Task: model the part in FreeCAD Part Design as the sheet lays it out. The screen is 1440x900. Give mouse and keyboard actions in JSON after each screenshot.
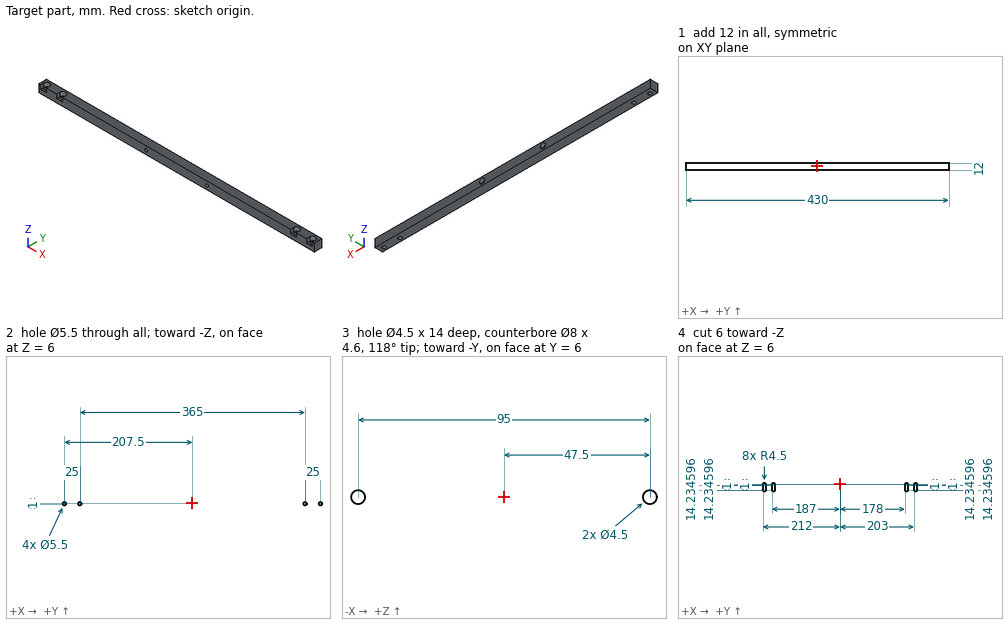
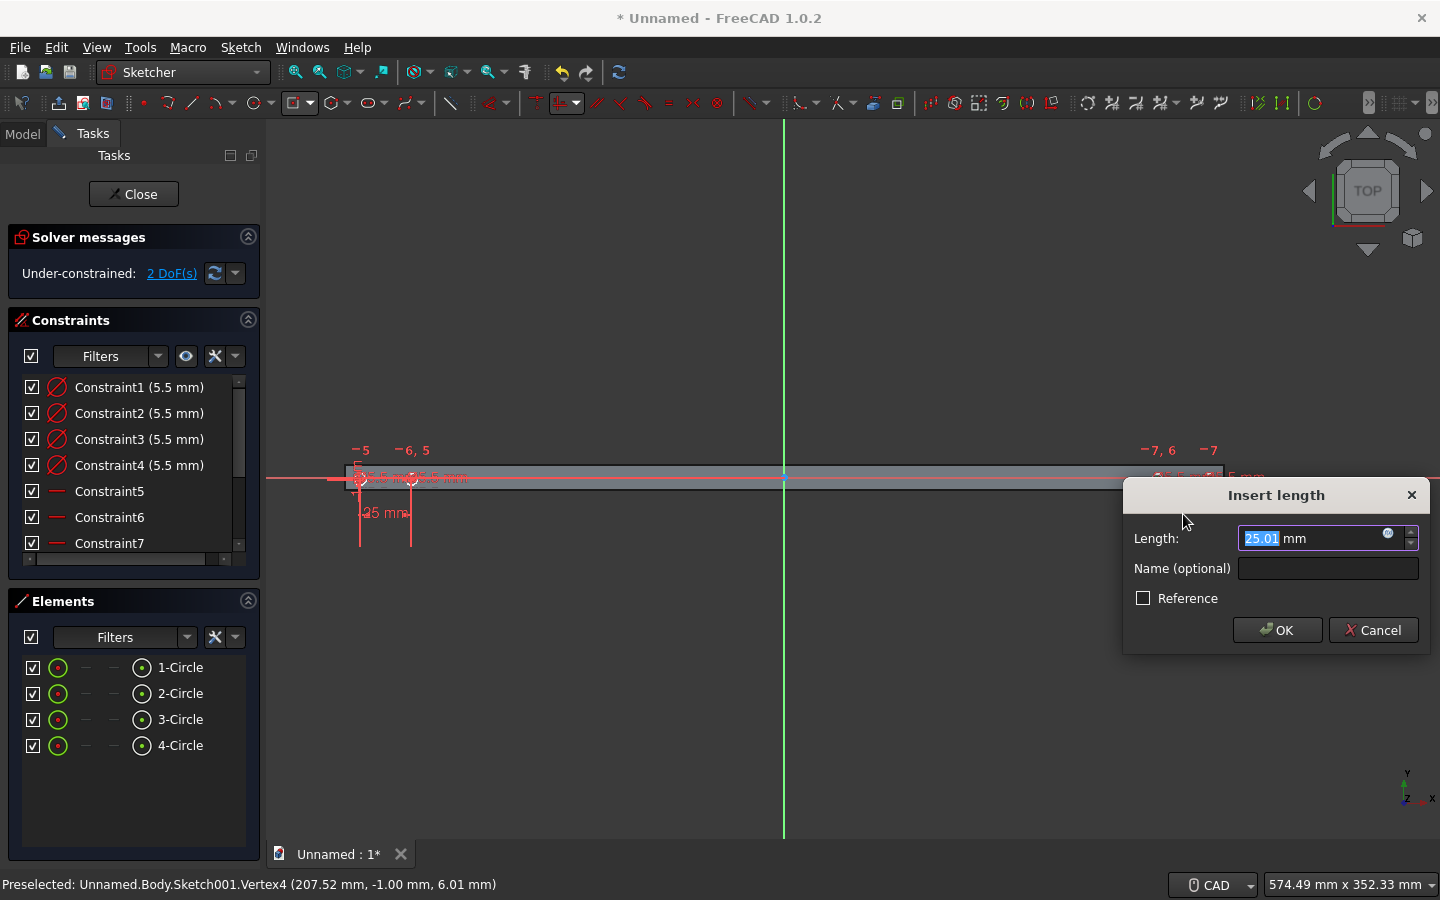
{"action": "type", "text": "25"}
{"action": "key", "text": "Return"}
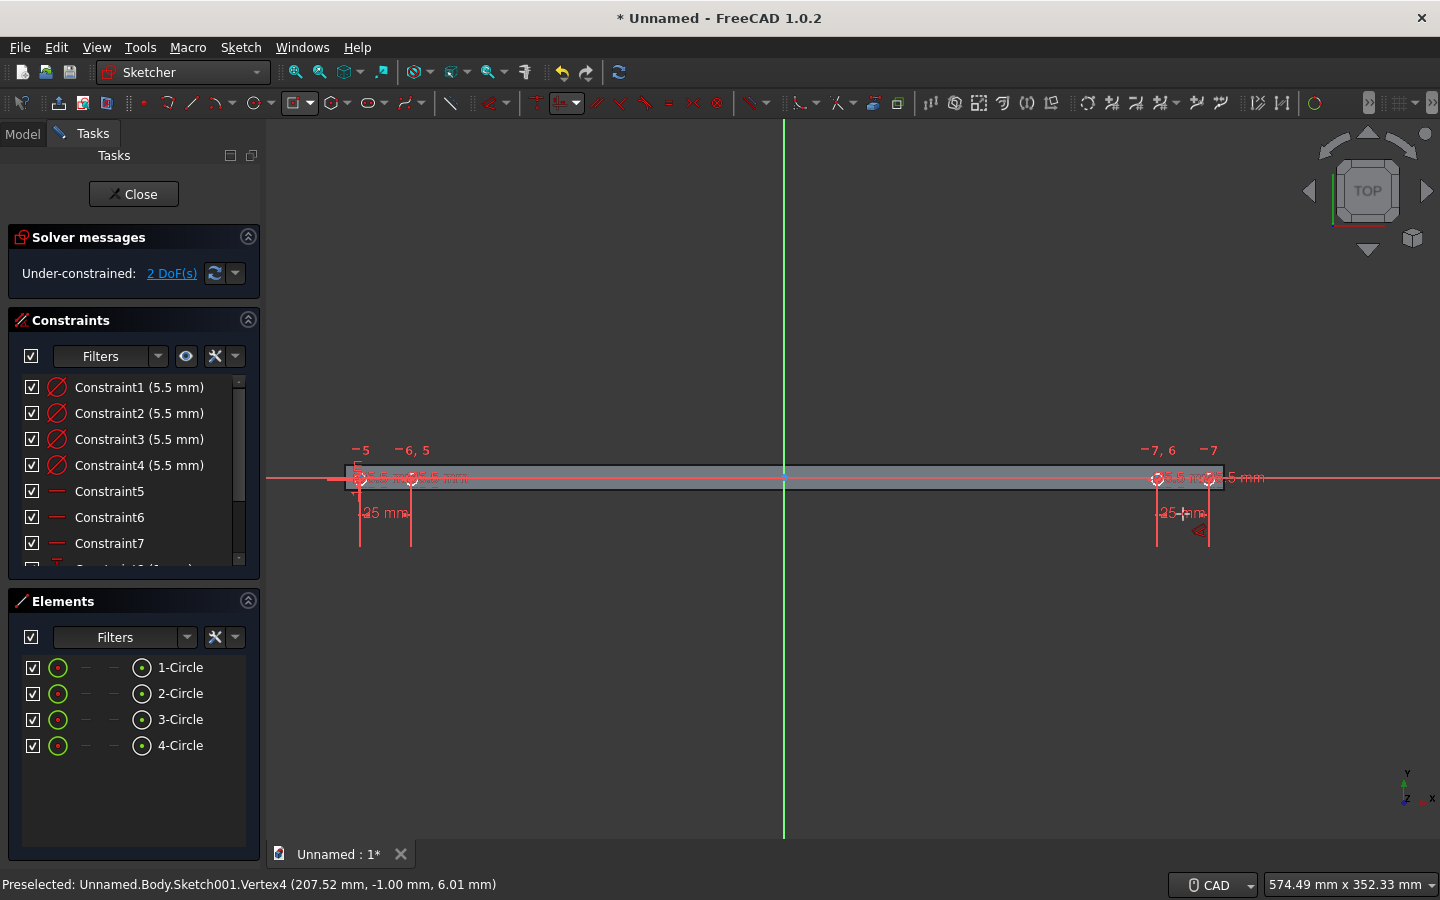
{"action": "left_click", "coordinate": [411, 480]}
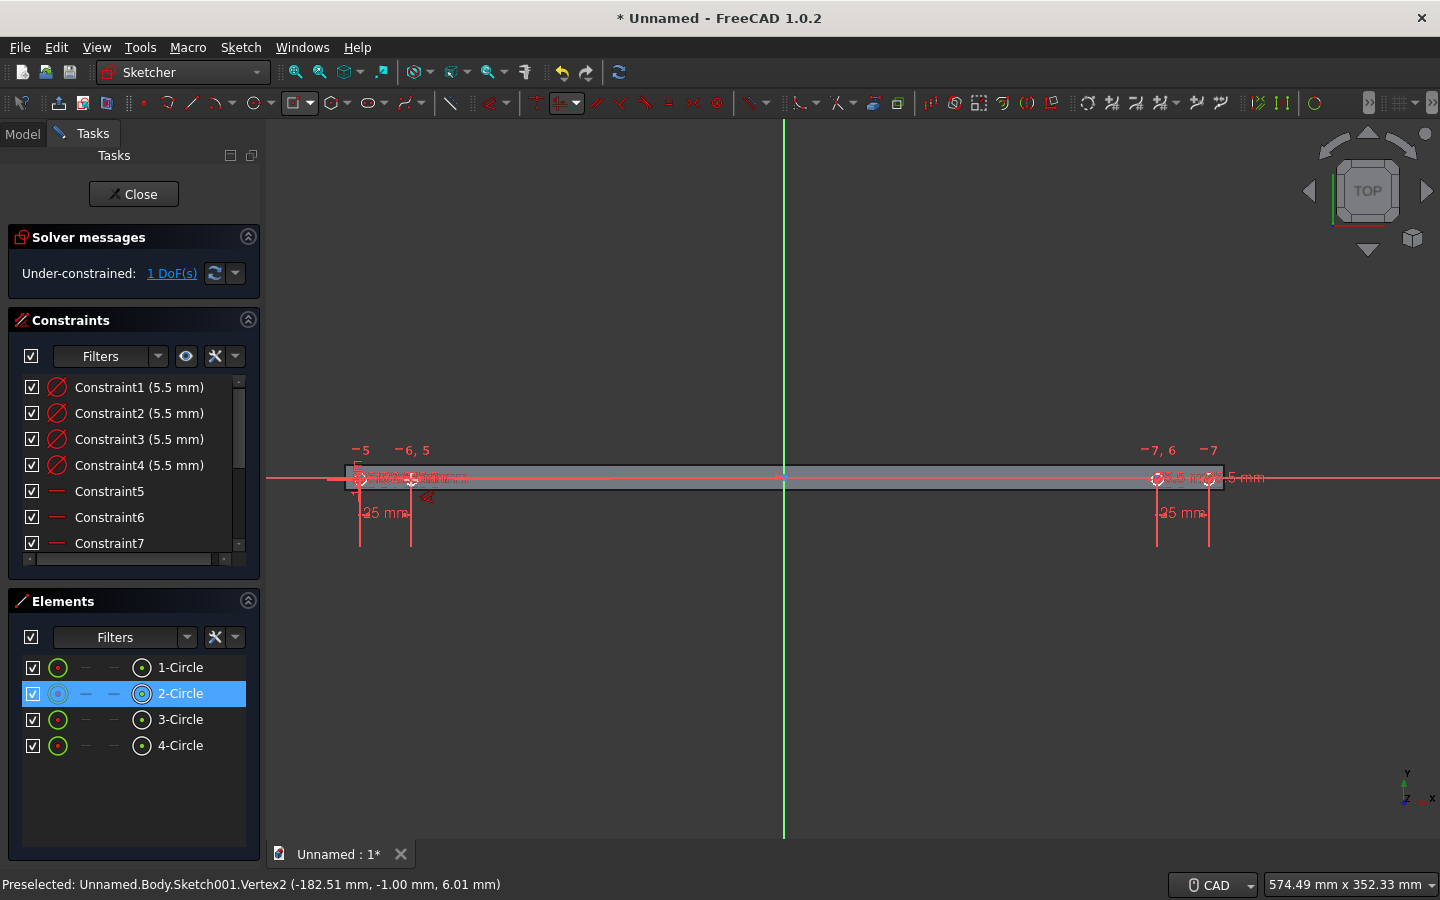
{"action": "left_click", "coordinate": [1157, 480]}
{"action": "left_click", "coordinate": [613, 514]}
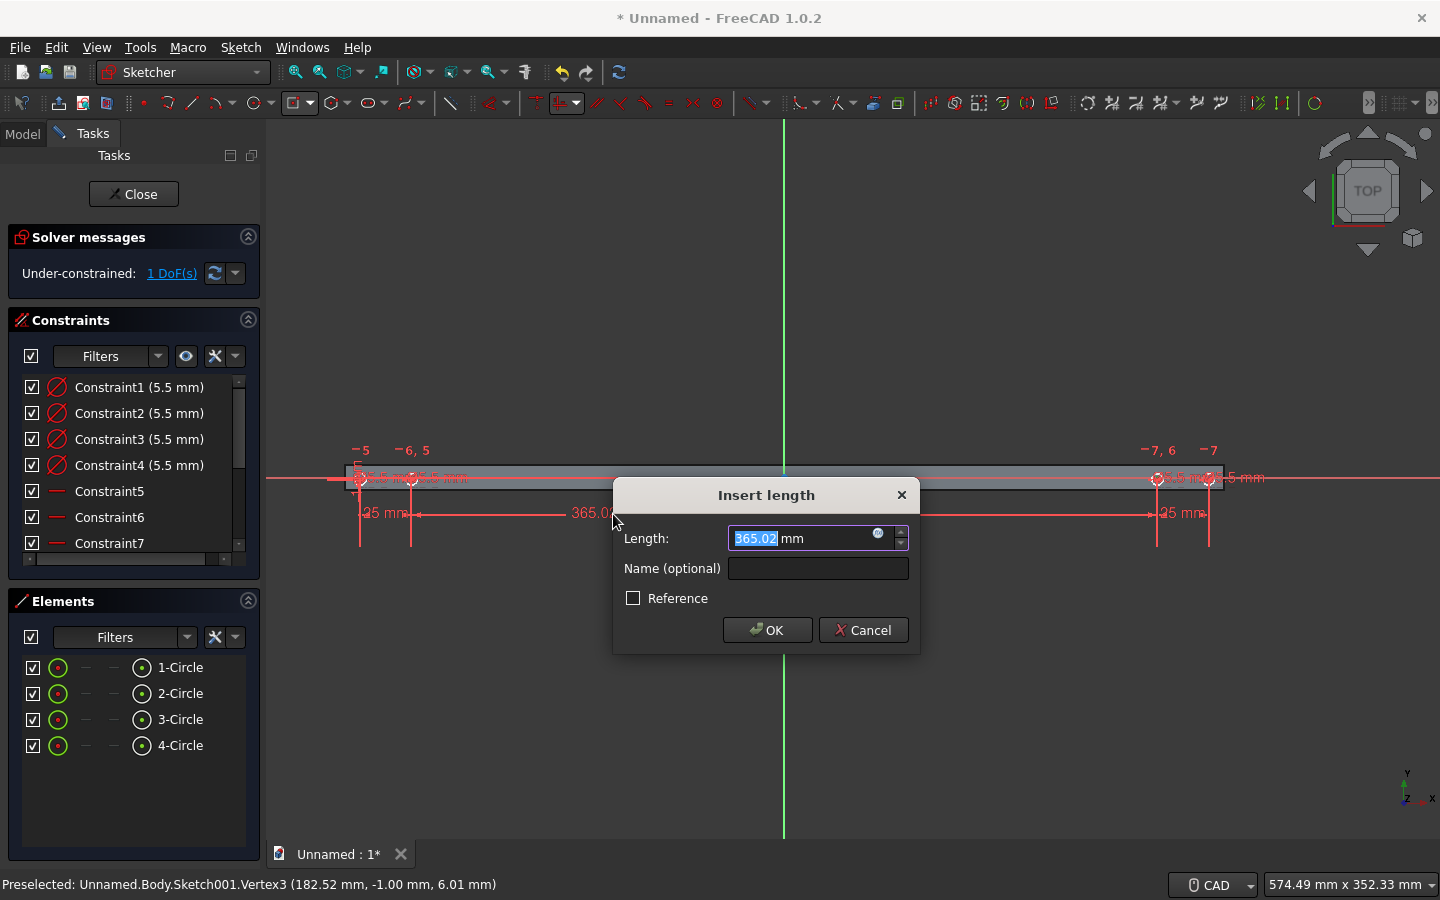
{"action": "type", "text": "365"}
{"action": "key", "text": "Return"}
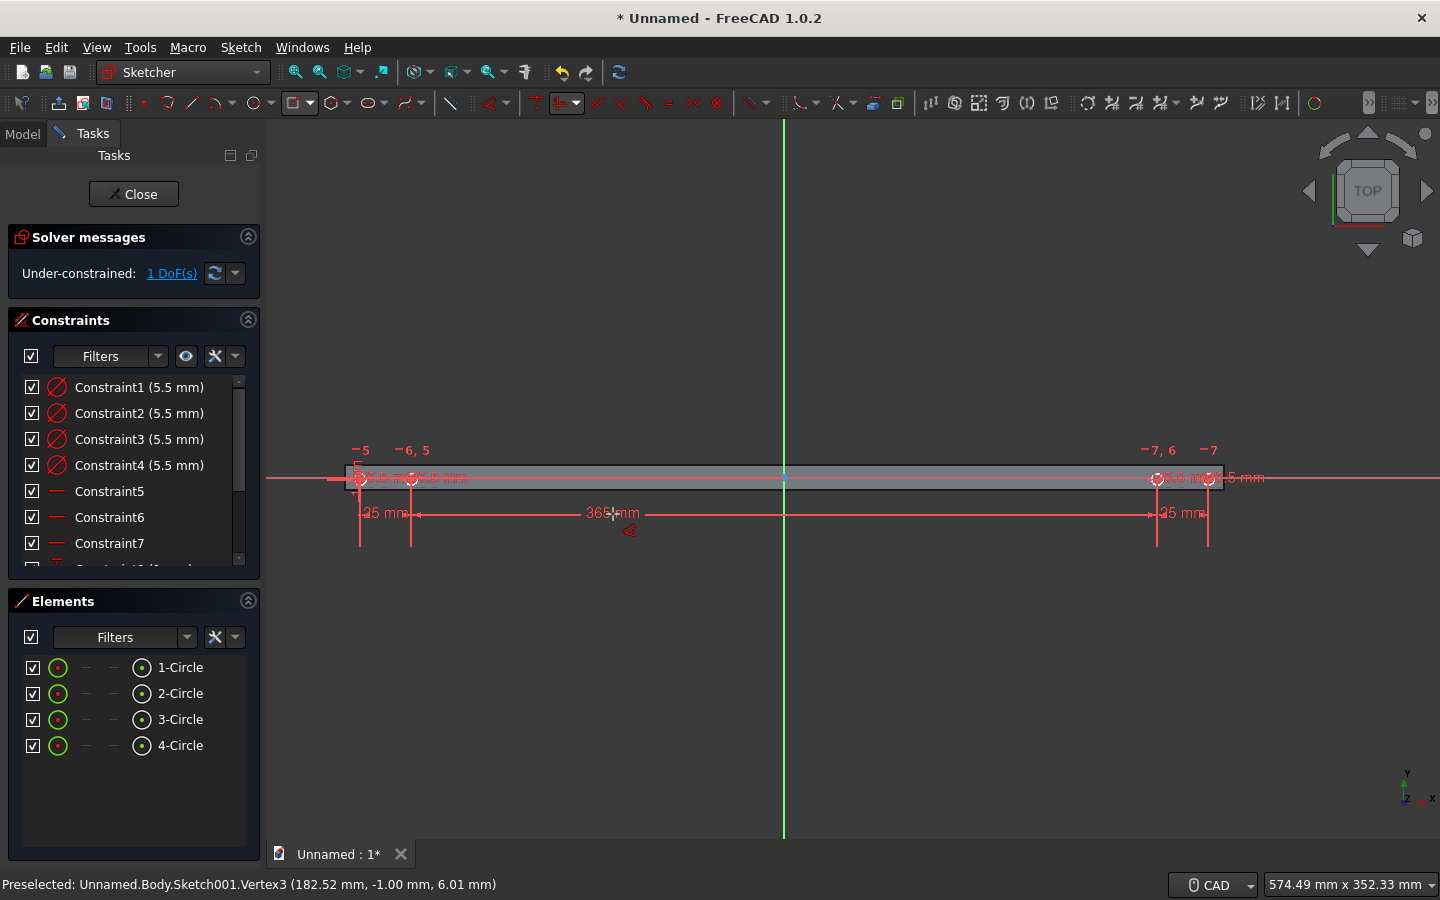
{"action": "left_click", "coordinate": [360, 480]}
{"action": "left_click", "coordinate": [572, 444]}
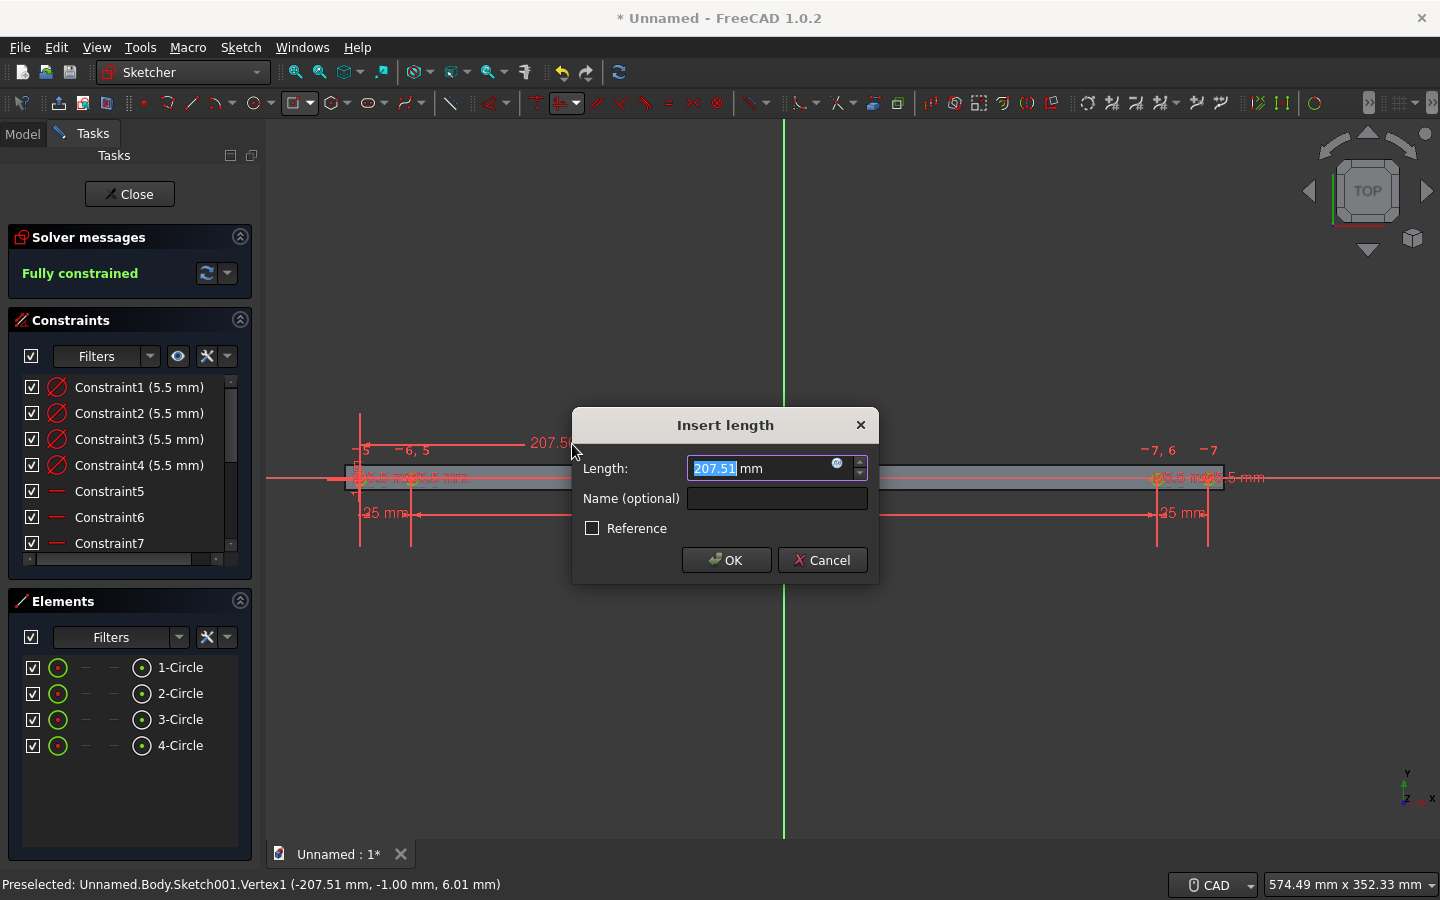
{"action": "type", "text": "207.5"}
{"action": "key", "text": "Return"}
{"action": "key", "text": "Escape"}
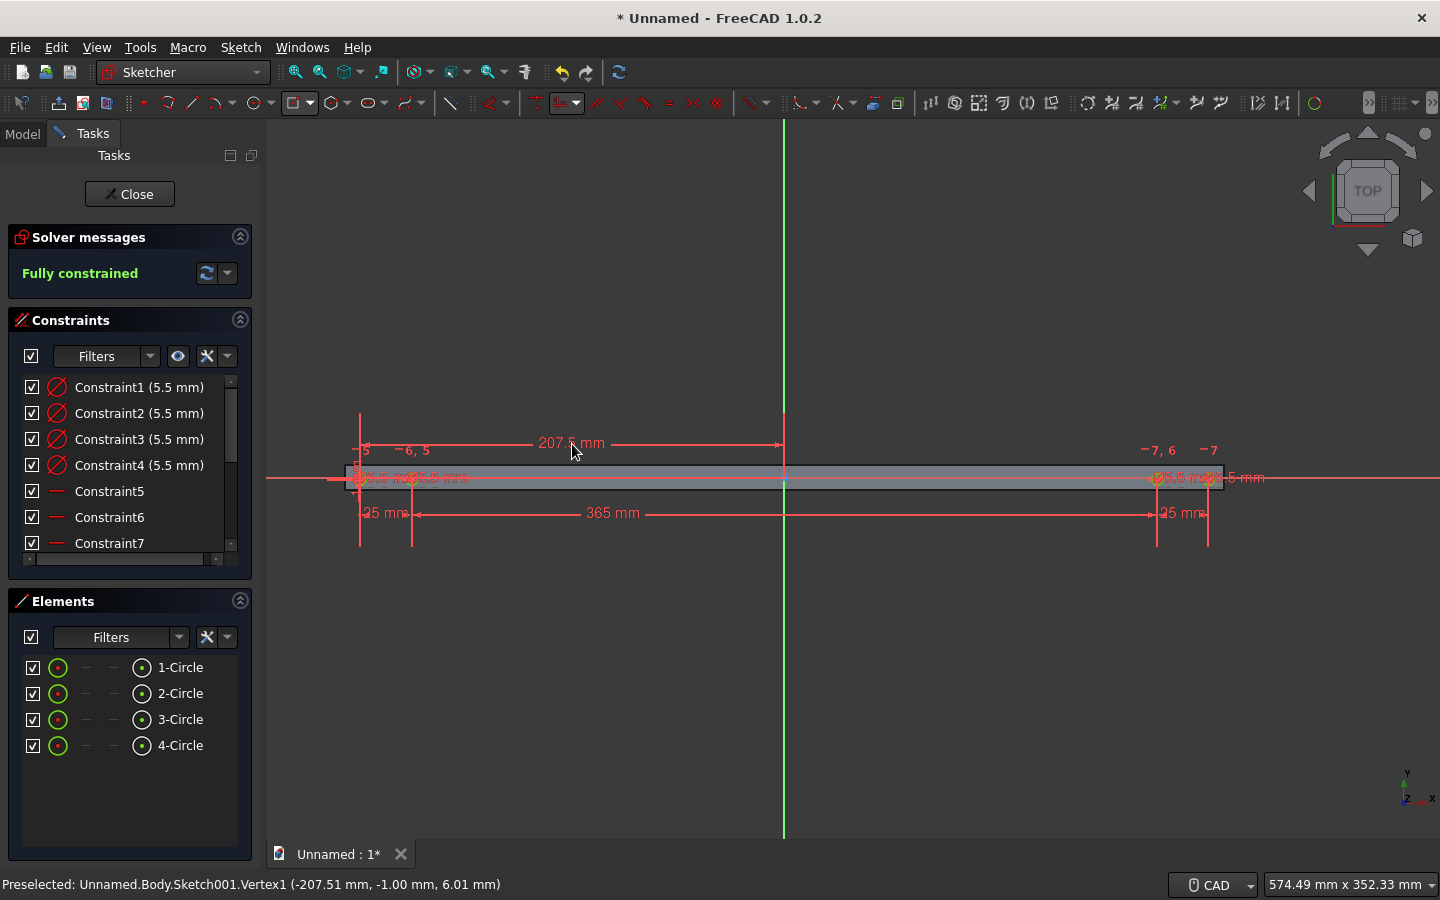
{"action": "left_click", "coordinate": [130, 194]}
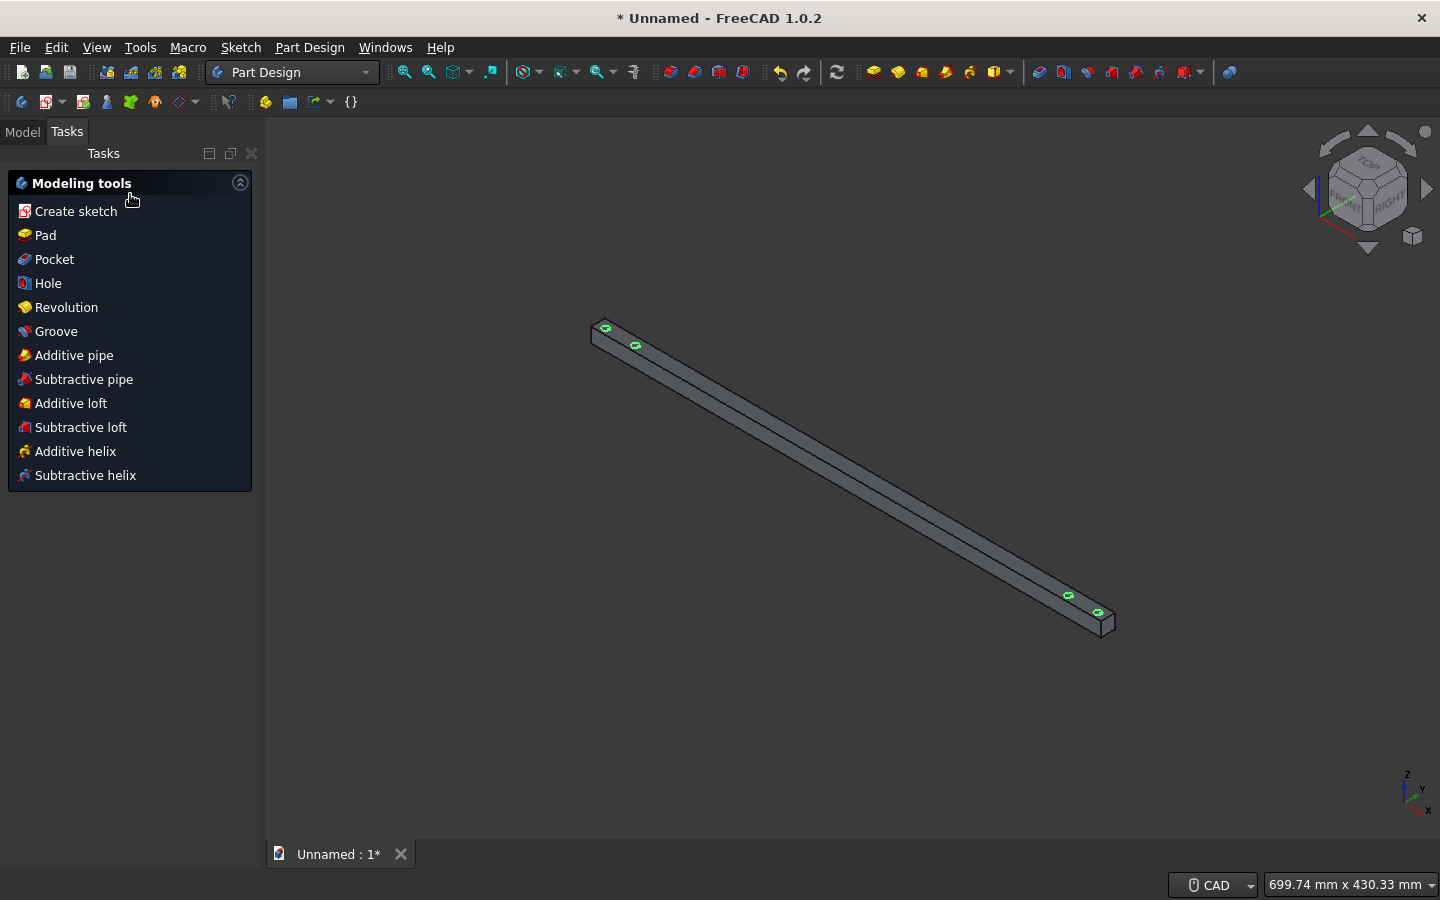
{"action": "left_click", "coordinate": [1064, 72]}